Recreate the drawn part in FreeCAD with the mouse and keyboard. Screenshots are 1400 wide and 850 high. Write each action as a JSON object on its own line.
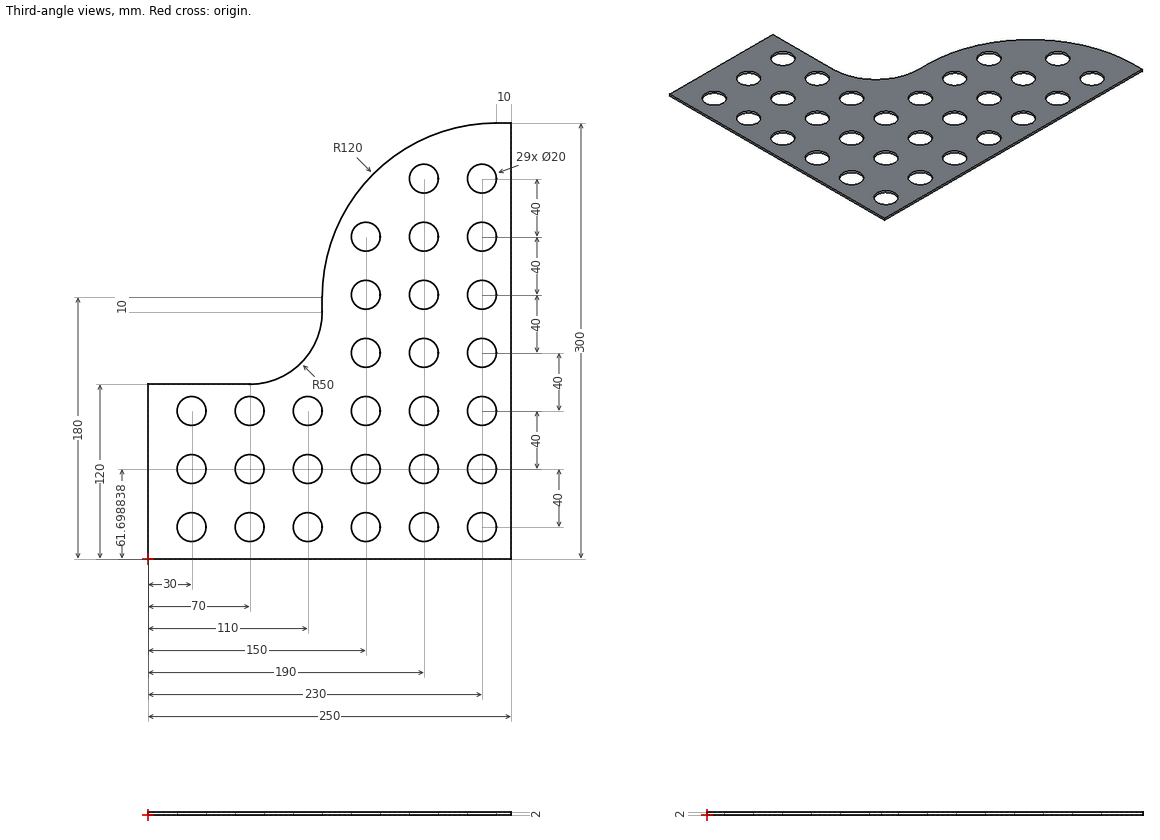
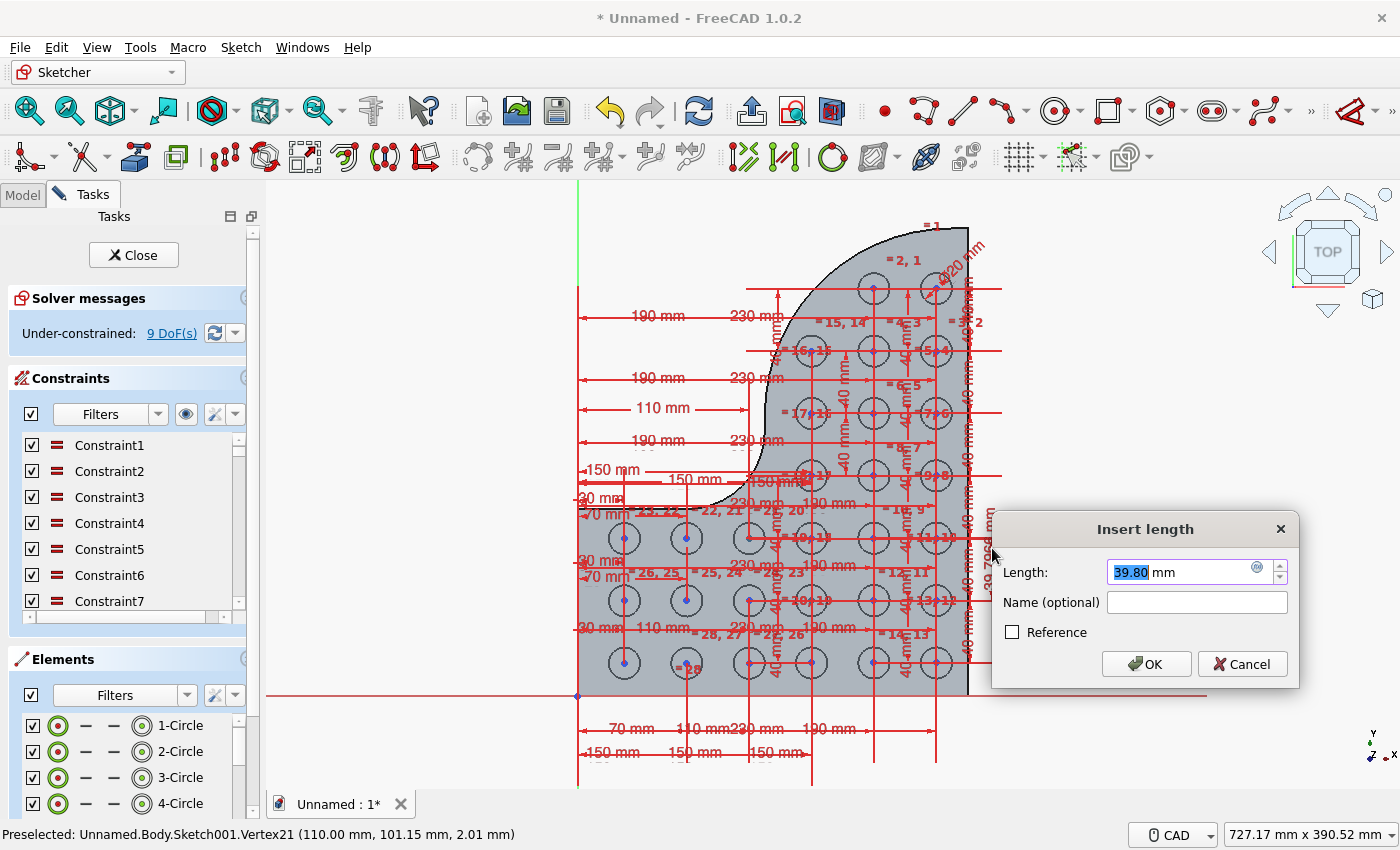
{"action": "type", "text": "40"}
{"action": "key", "text": "Return"}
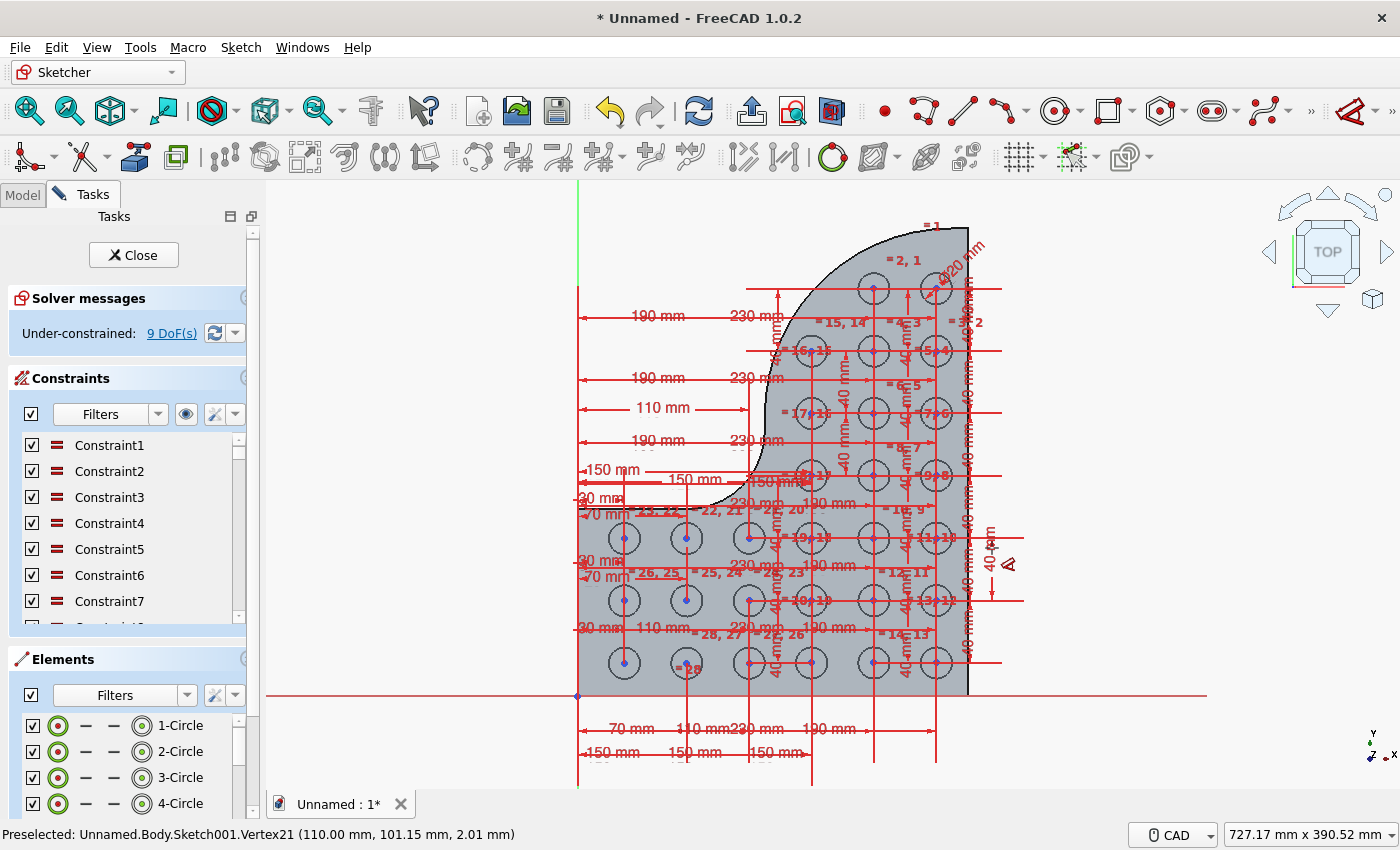
{"action": "left_click", "coordinate": [812, 601]}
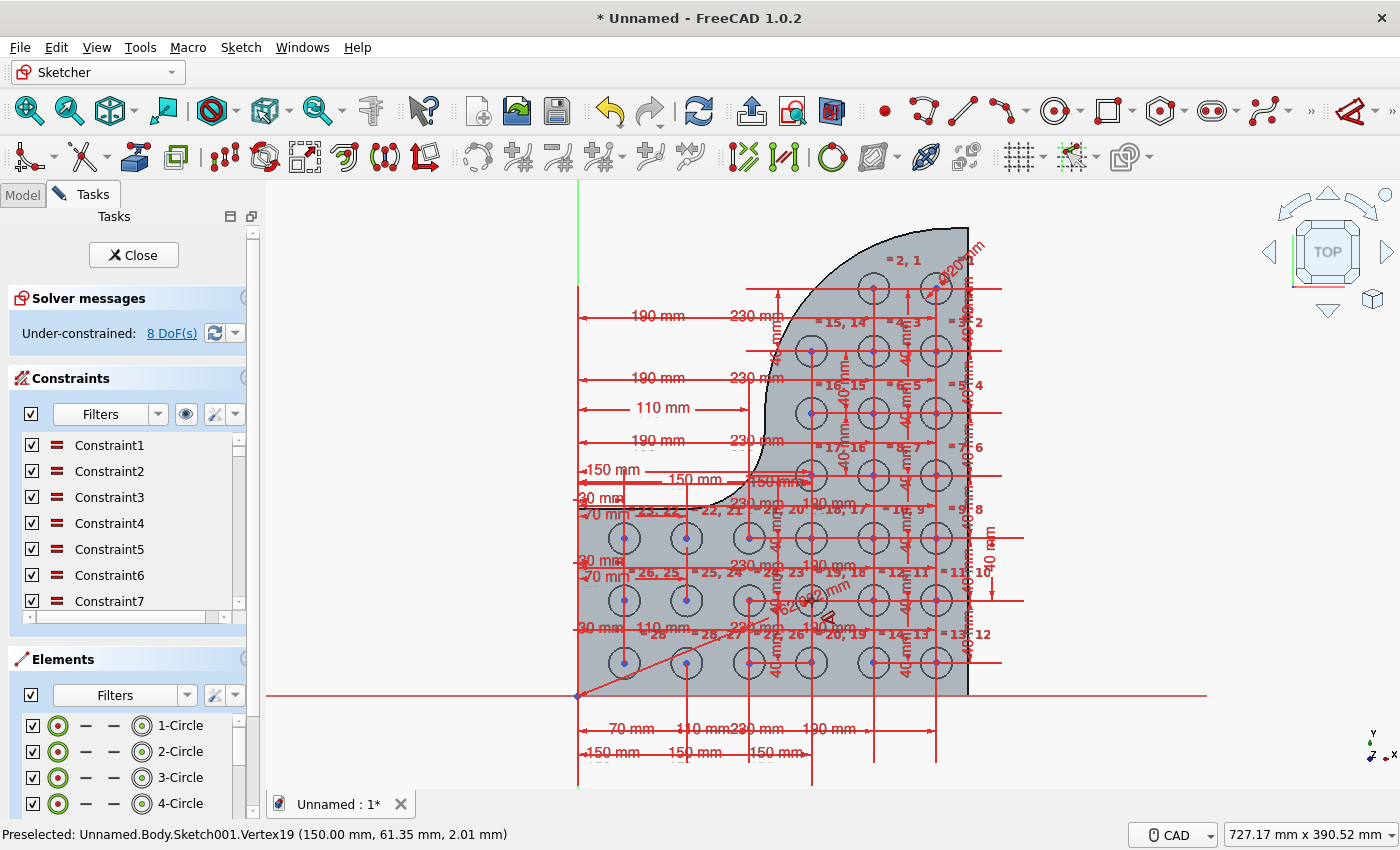
{"action": "left_click", "coordinate": [687, 539]}
{"action": "left_click", "coordinate": [533, 584]}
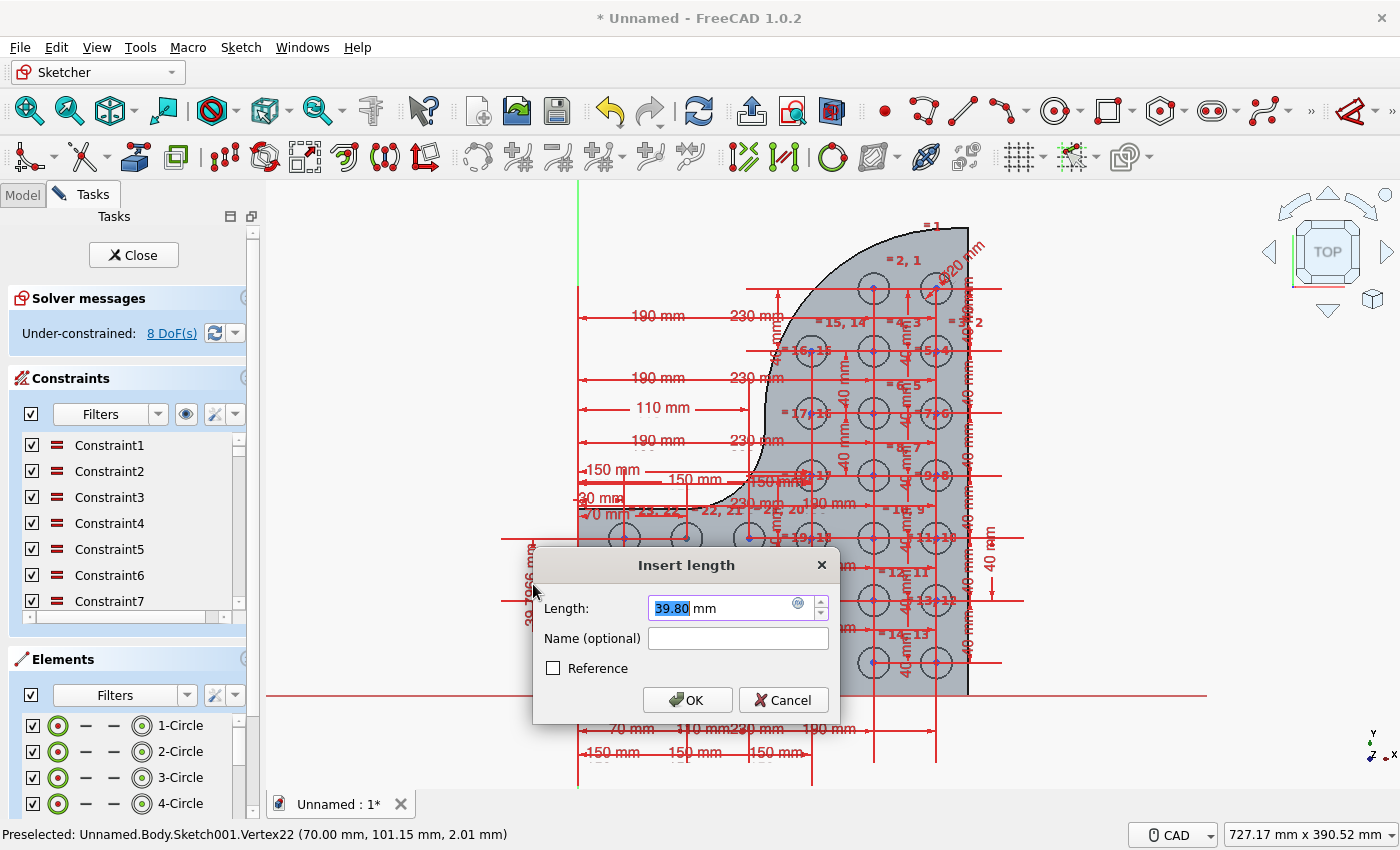
{"action": "type", "text": "40"}
{"action": "key", "text": "Return"}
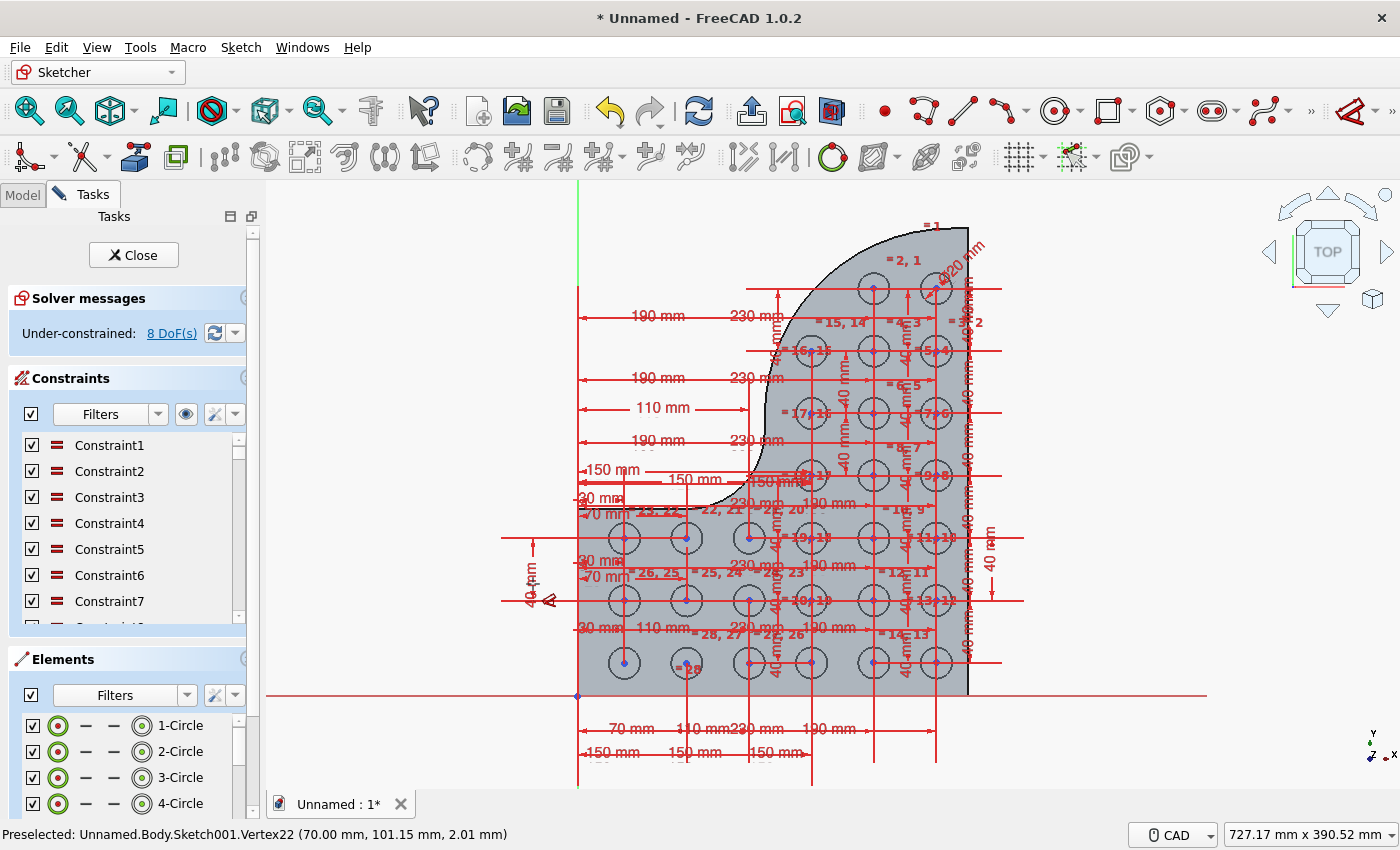
{"action": "left_click", "coordinate": [812, 476]}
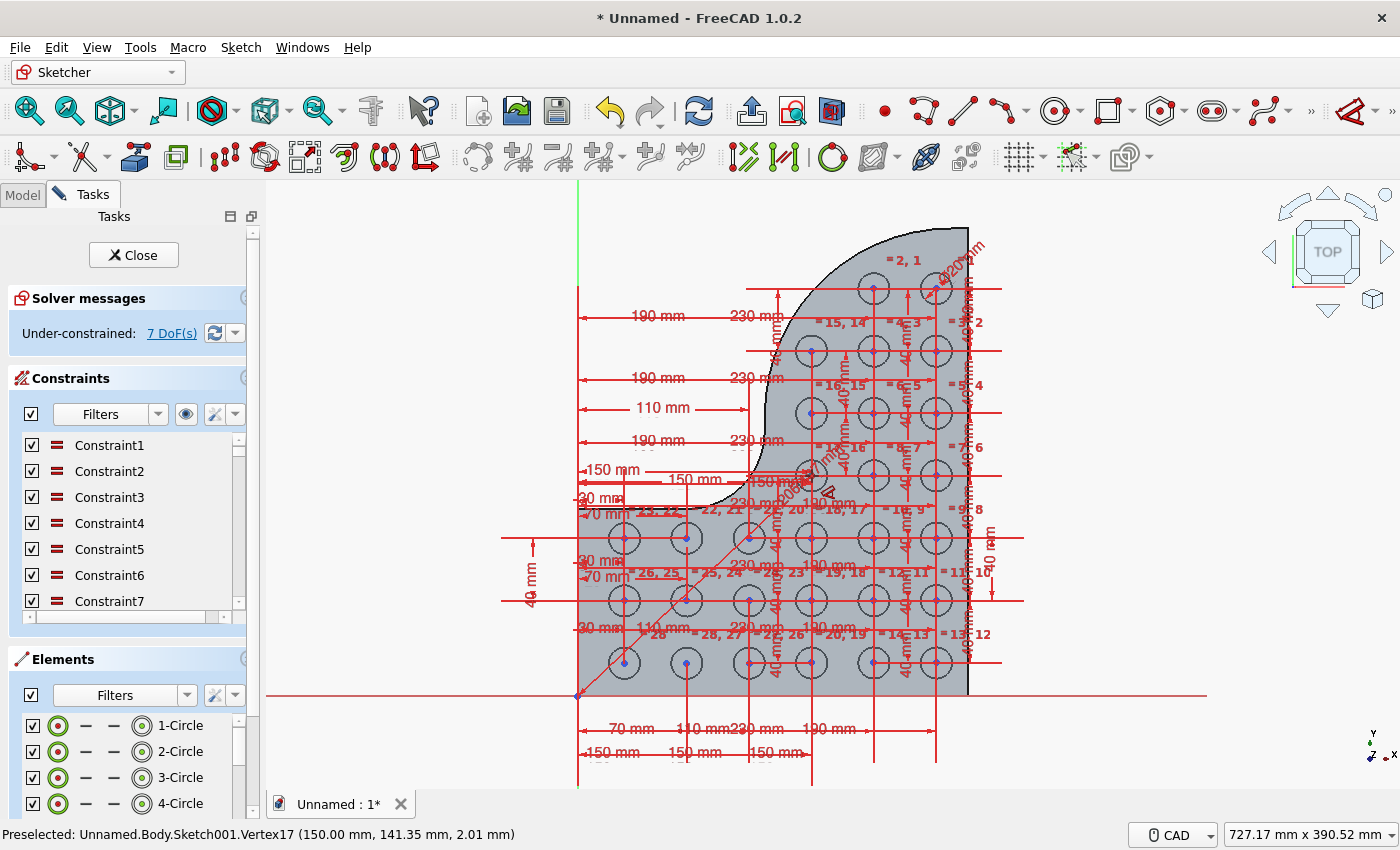
{"action": "left_click", "coordinate": [624, 539]}
{"action": "left_click", "coordinate": [518, 507]}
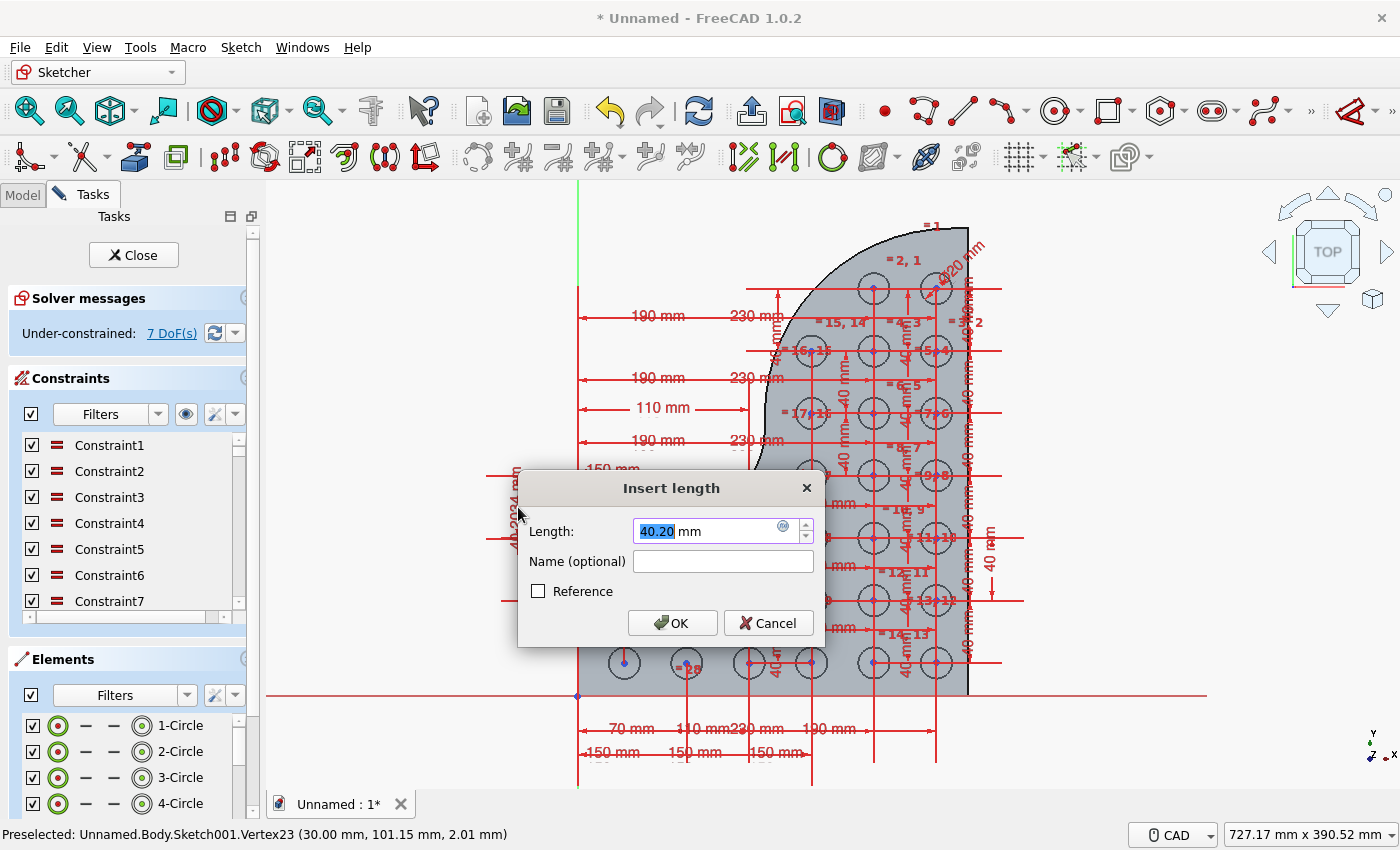
{"action": "type", "text": "40"}
{"action": "key", "text": "Return"}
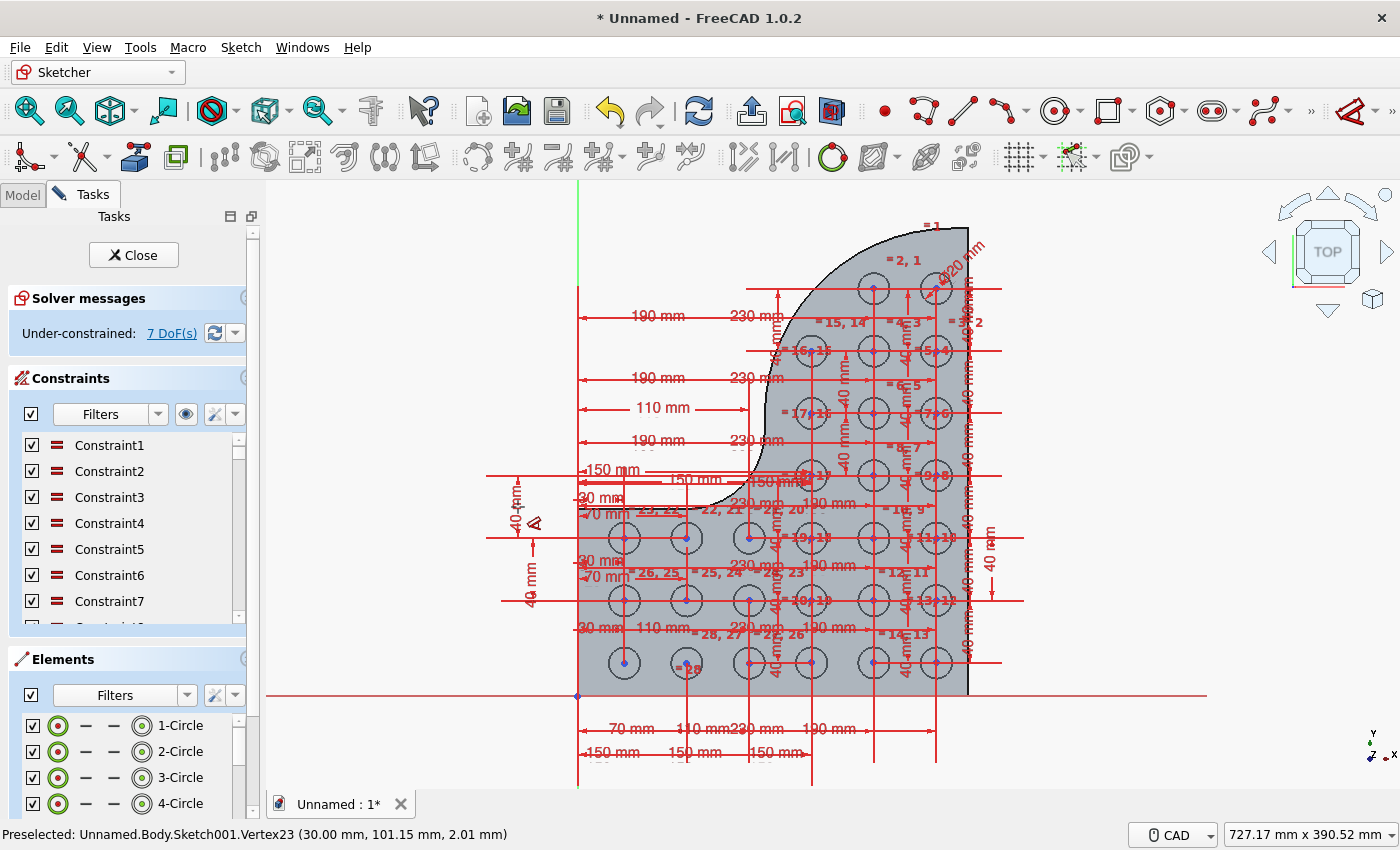
{"action": "left_click", "coordinate": [749, 538]}